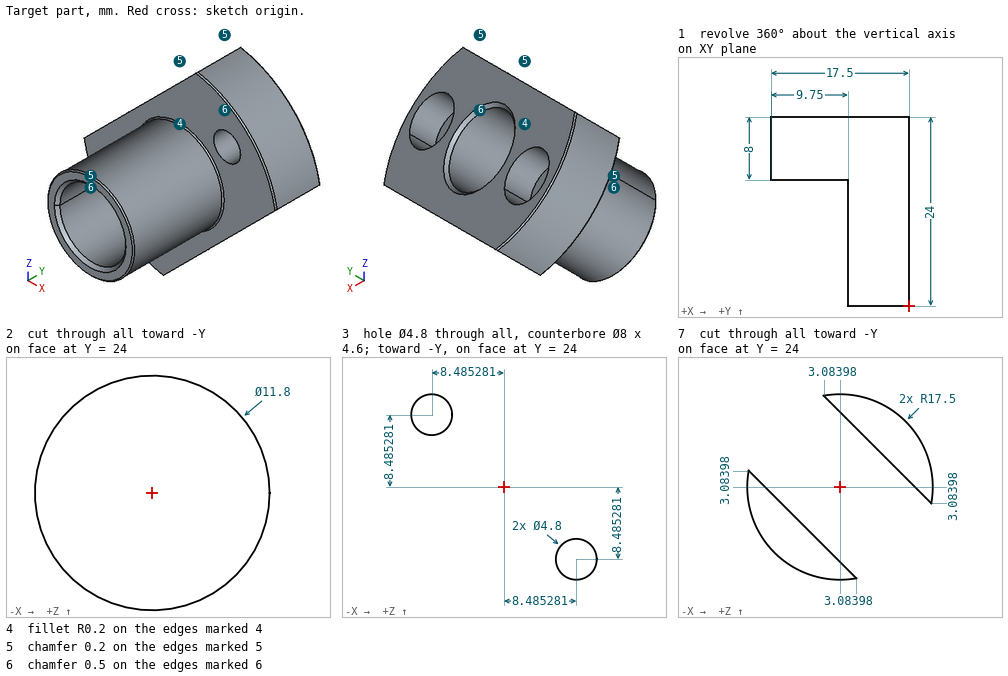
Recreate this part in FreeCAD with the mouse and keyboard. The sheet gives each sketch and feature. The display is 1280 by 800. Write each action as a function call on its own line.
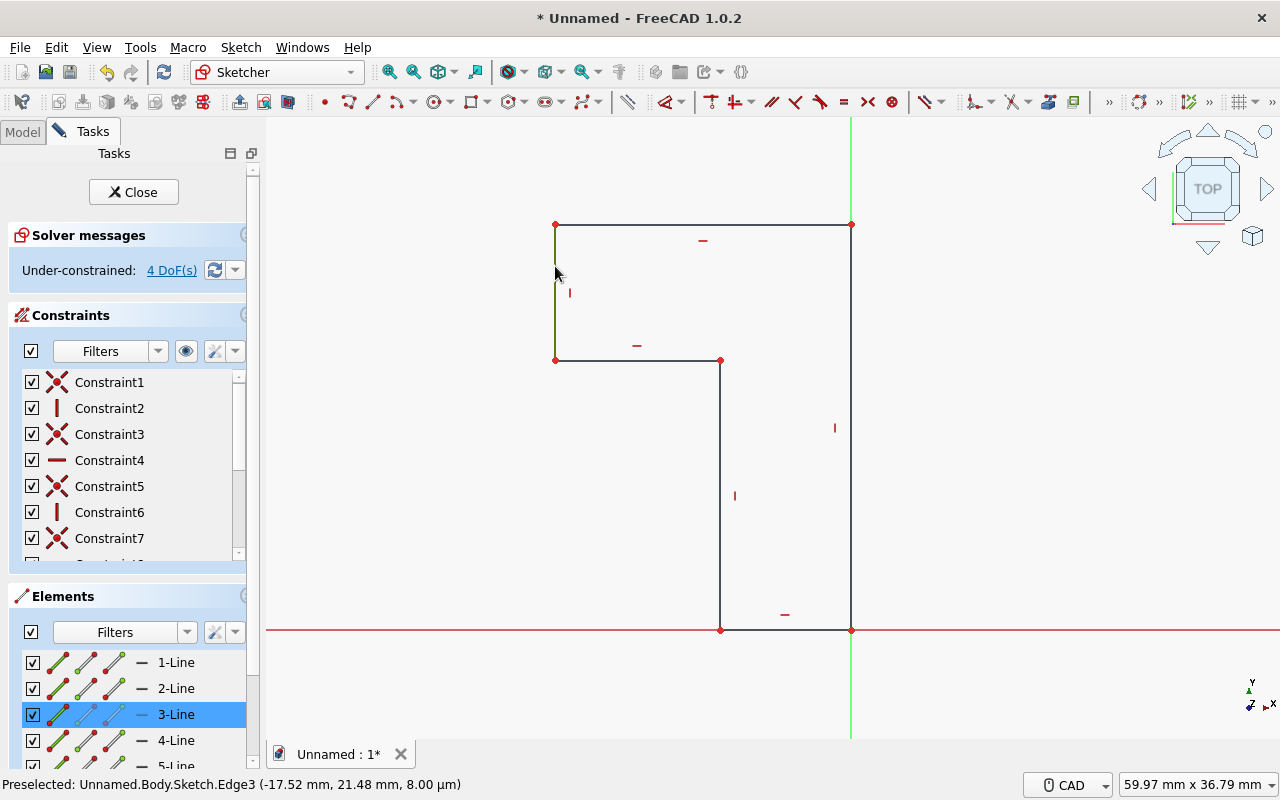
key(i)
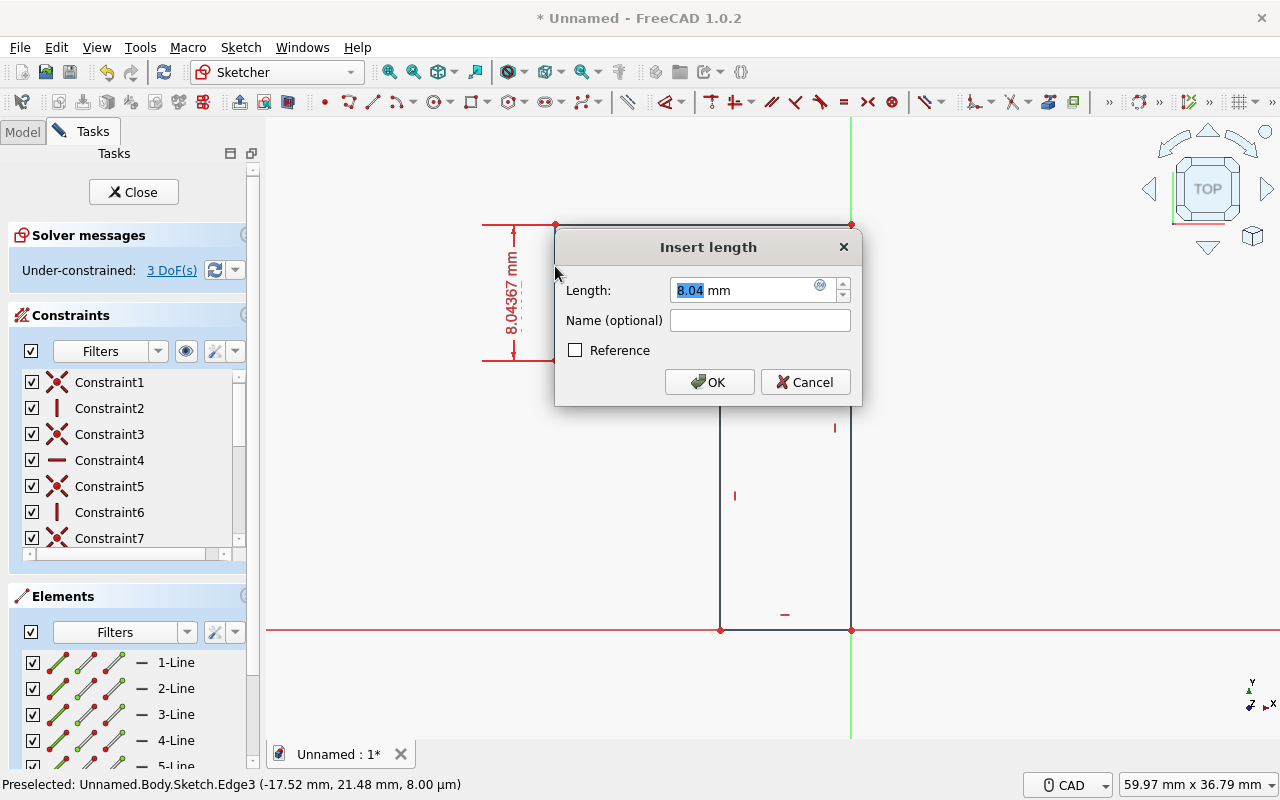
text(8)
key(Return)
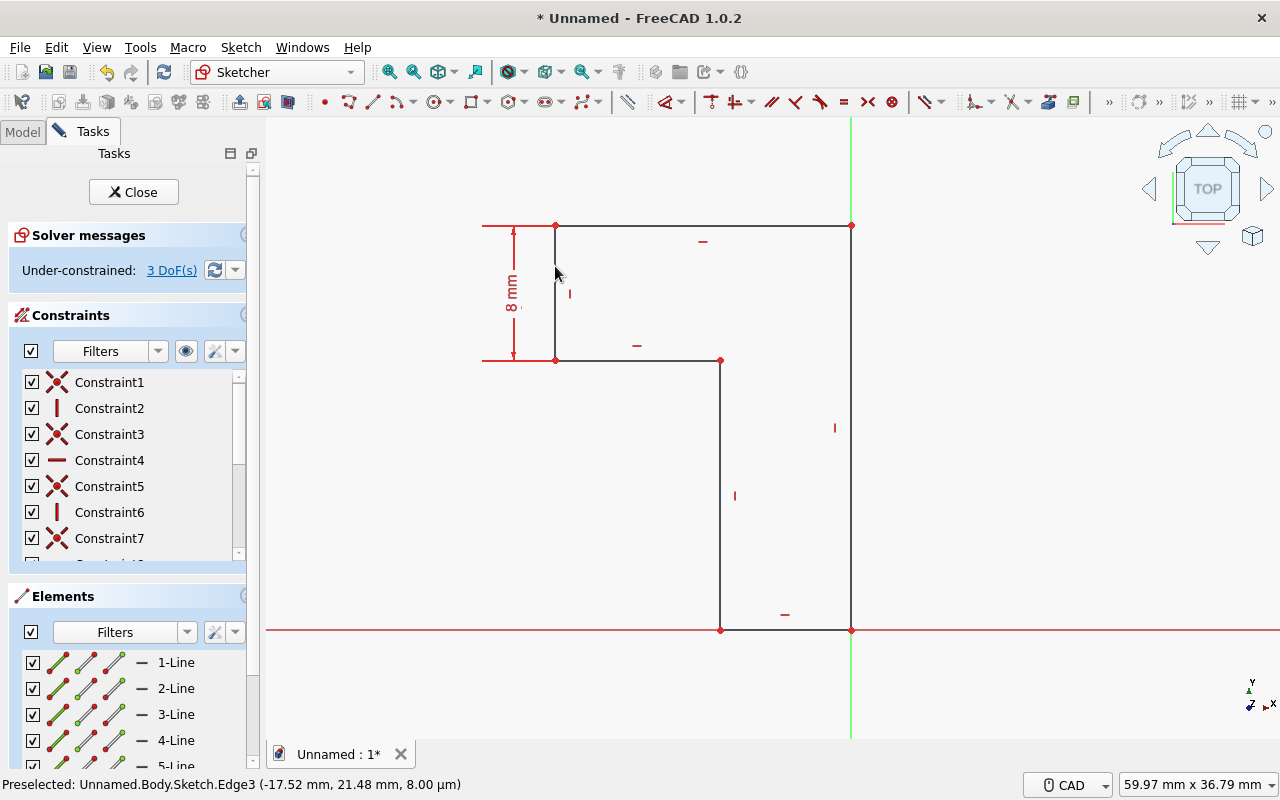
click(851, 509)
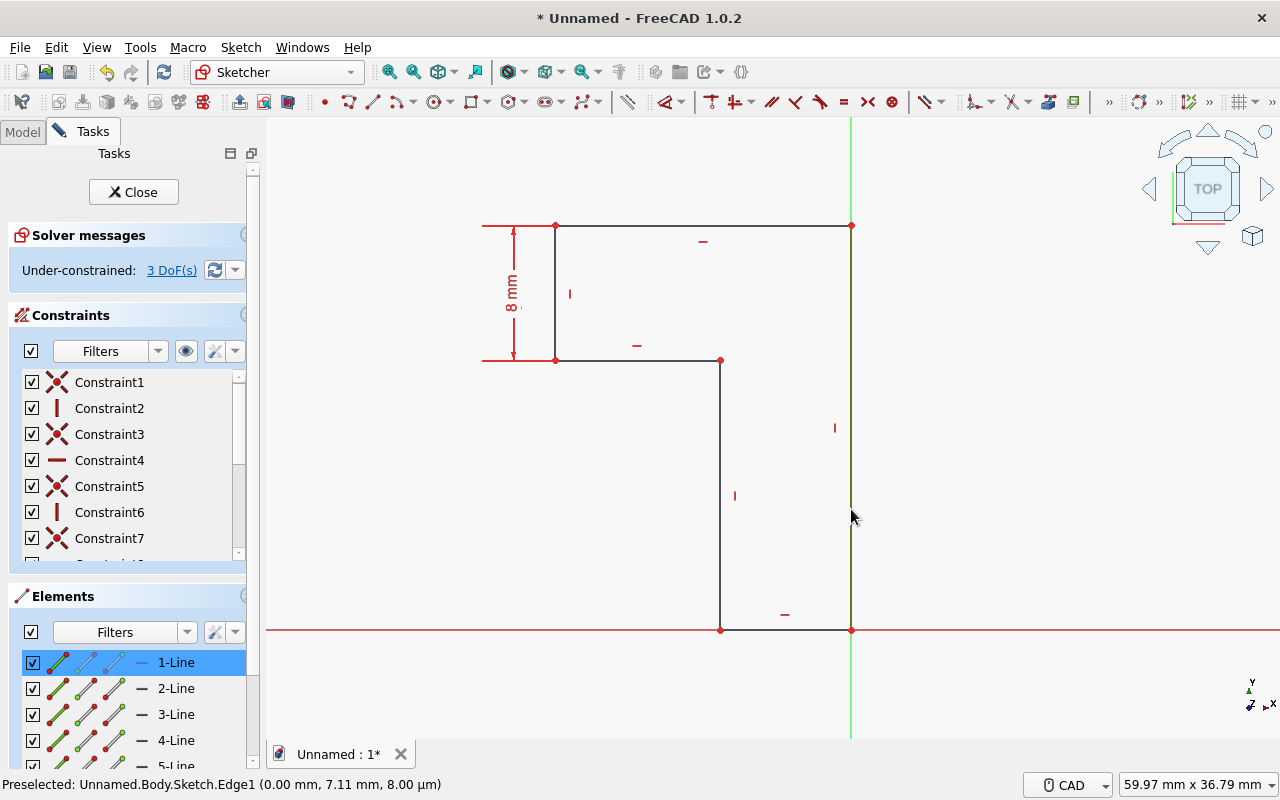
key(i)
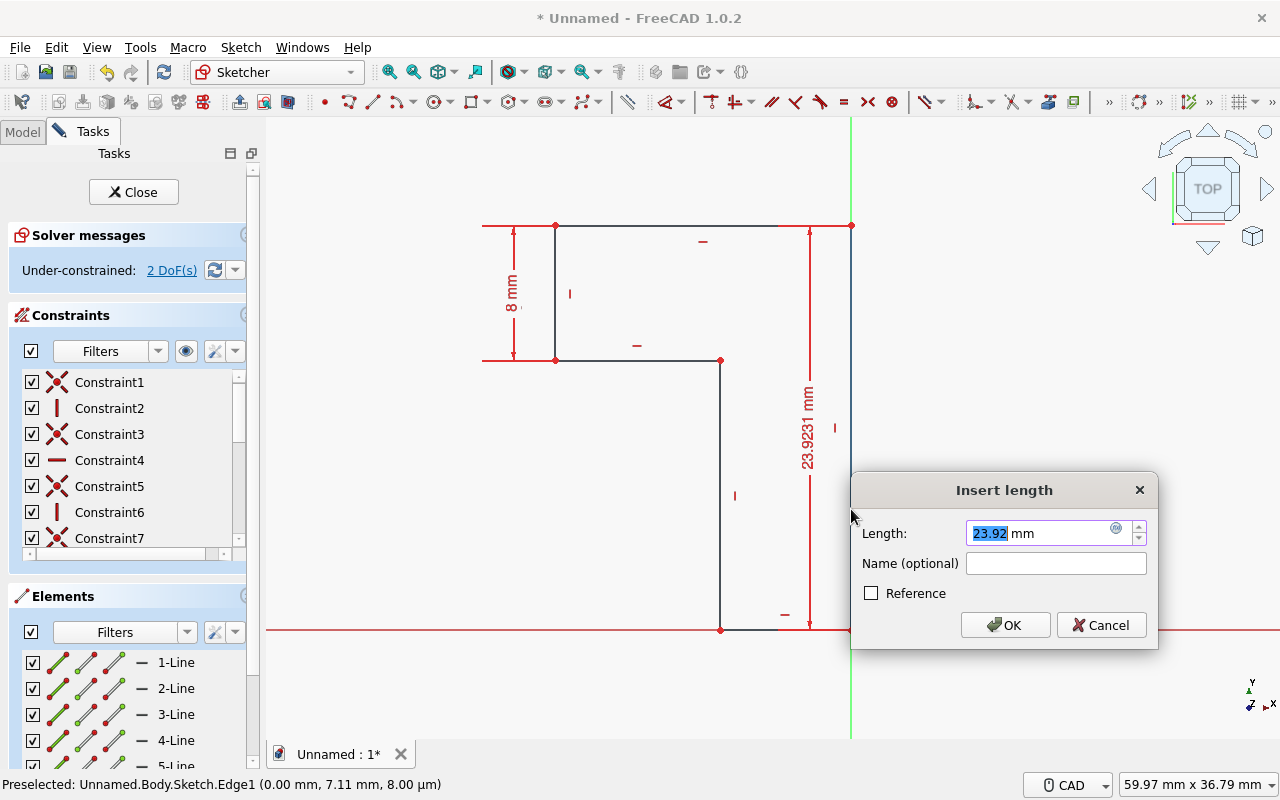
text(24)
key(Return)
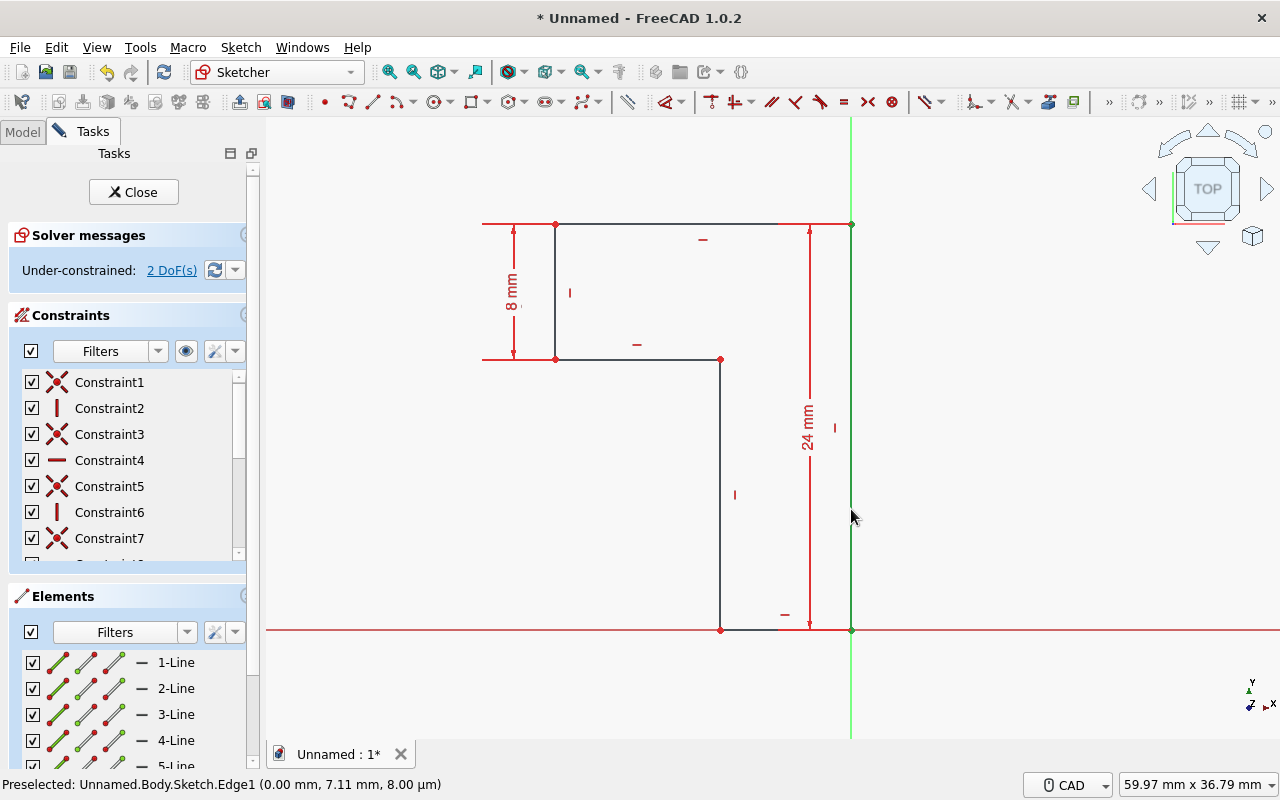
click(762, 224)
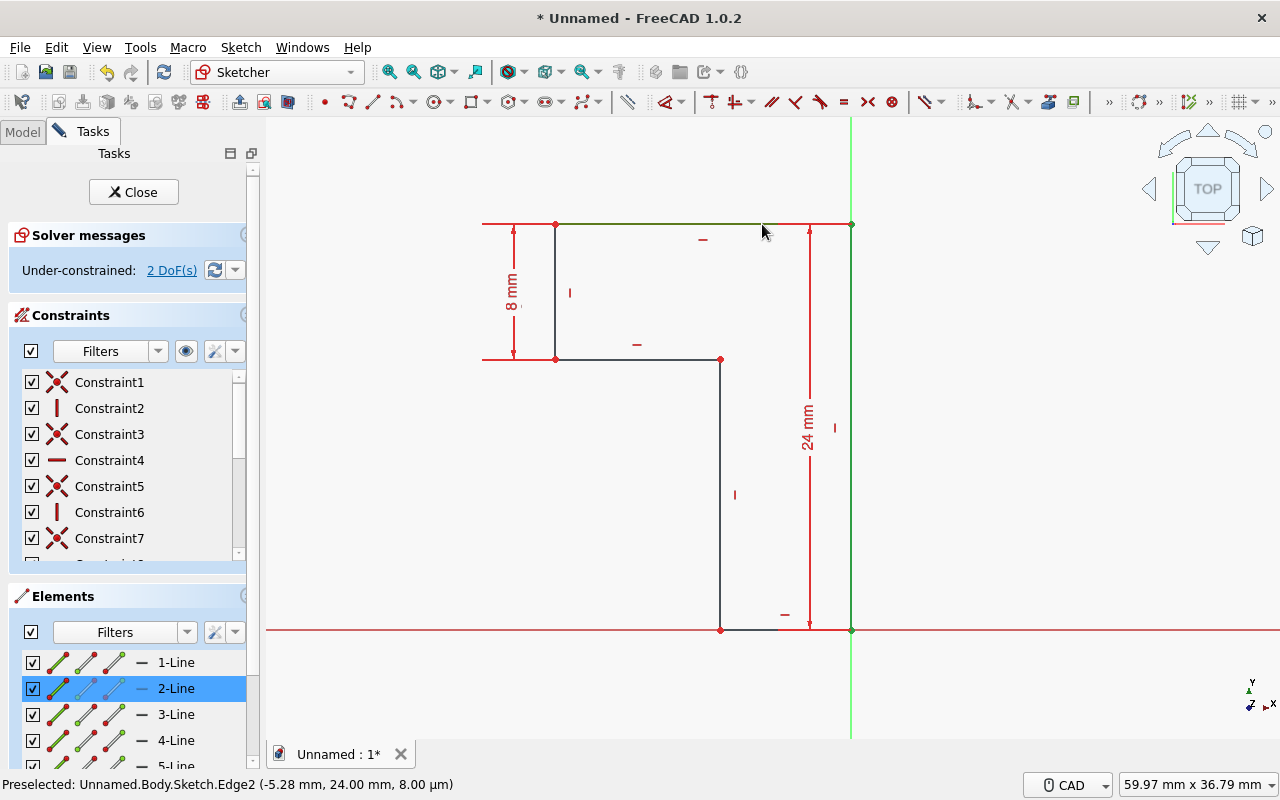
click(684, 102)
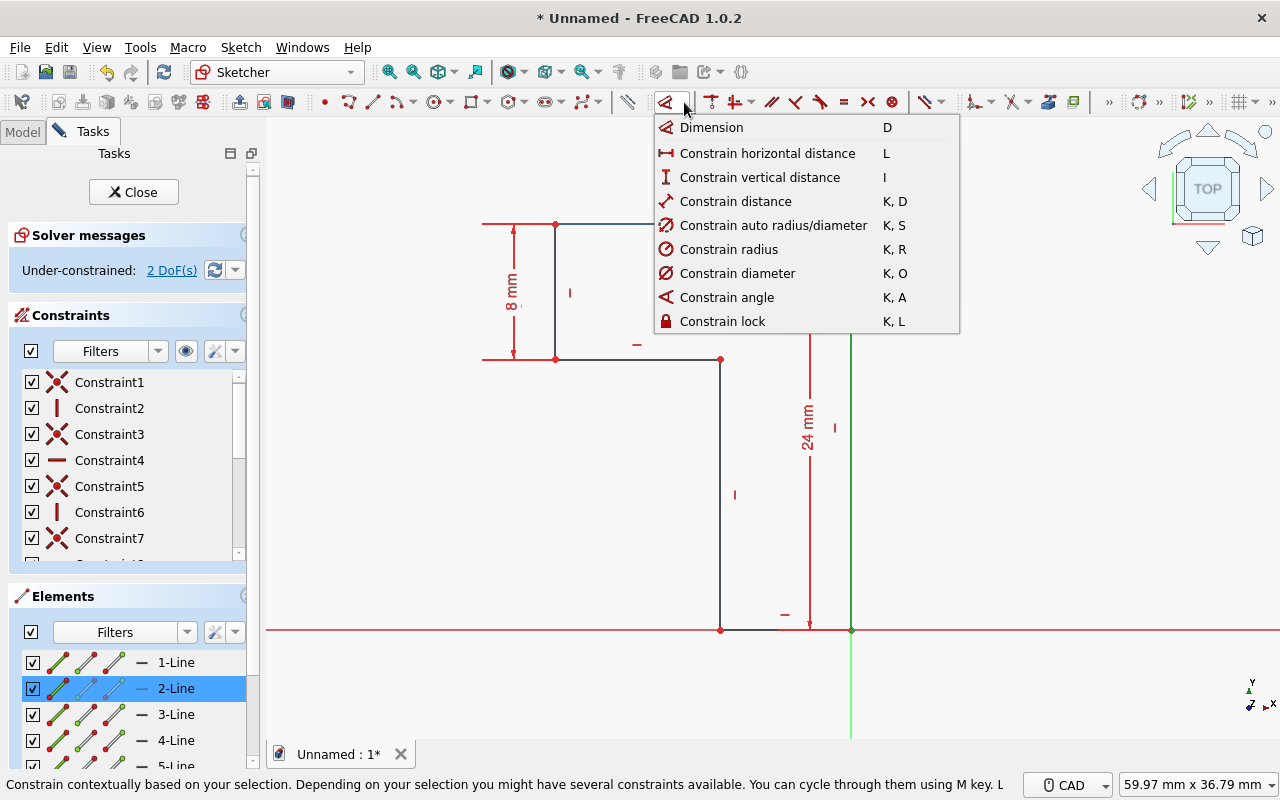
click(807, 153)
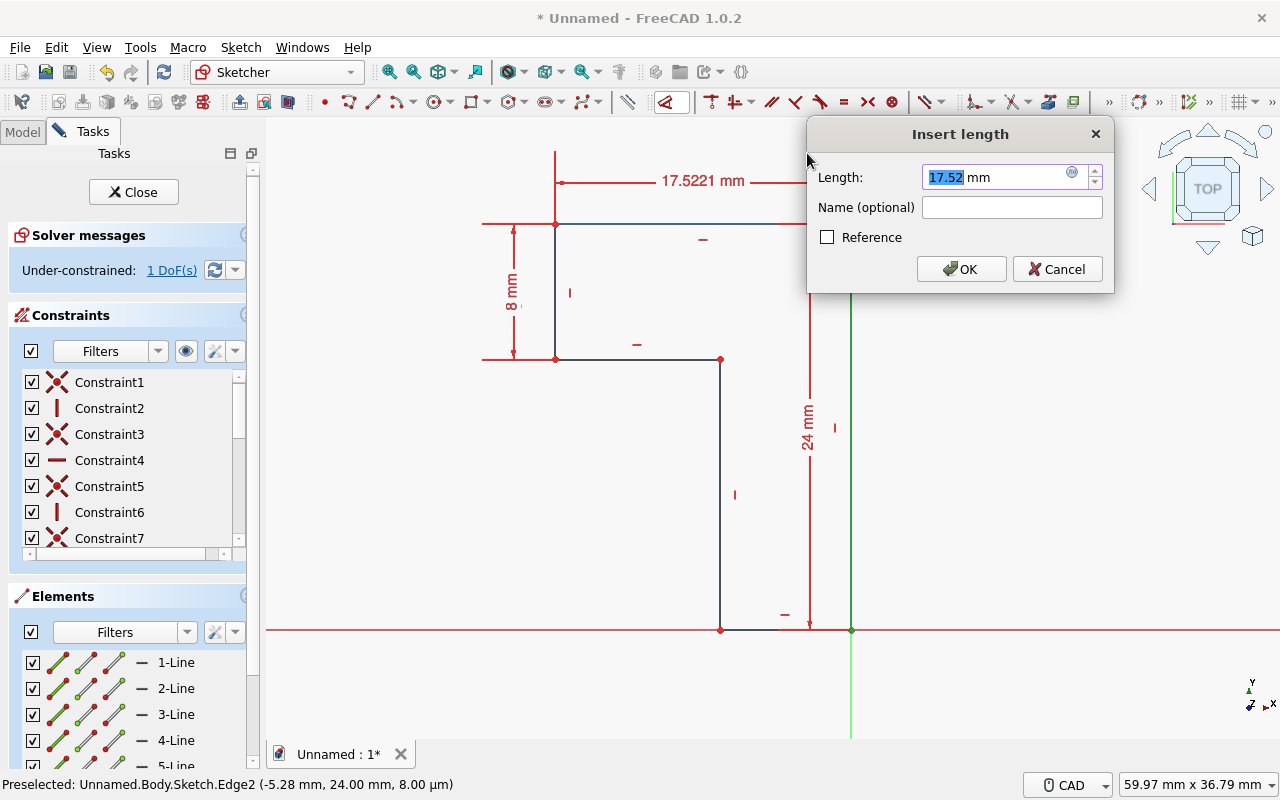
text(17.5)
key(Return)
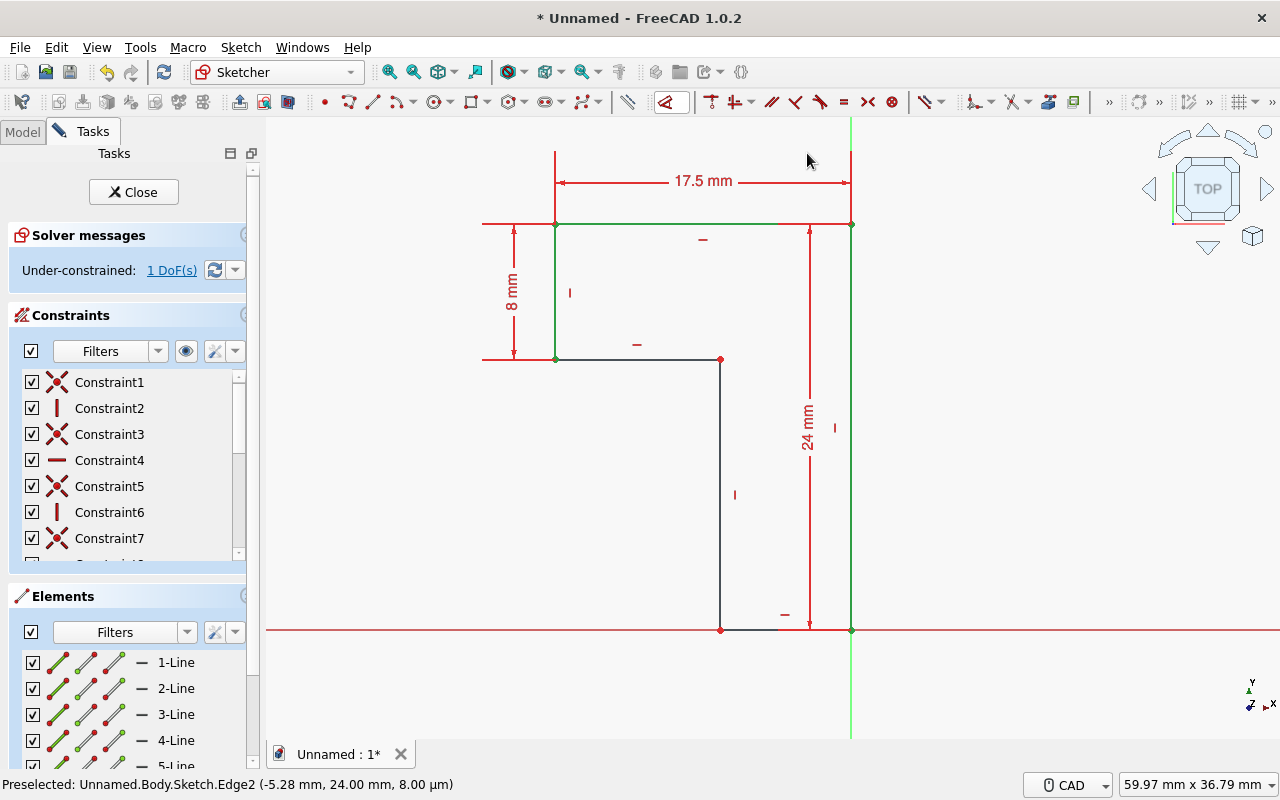
click(605, 360)